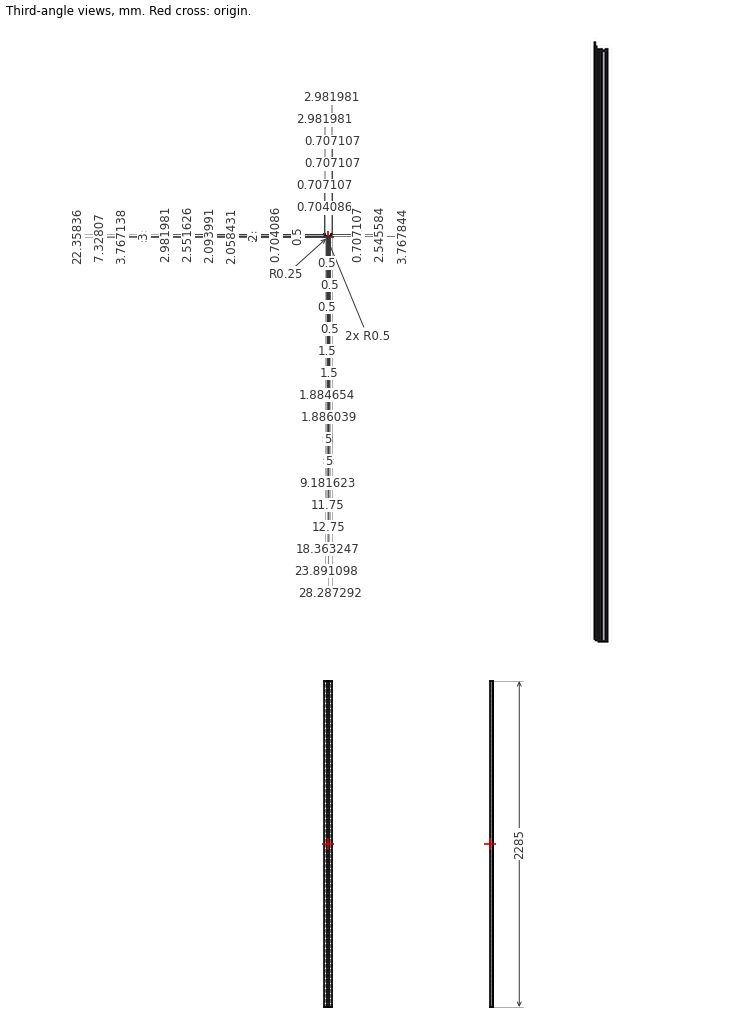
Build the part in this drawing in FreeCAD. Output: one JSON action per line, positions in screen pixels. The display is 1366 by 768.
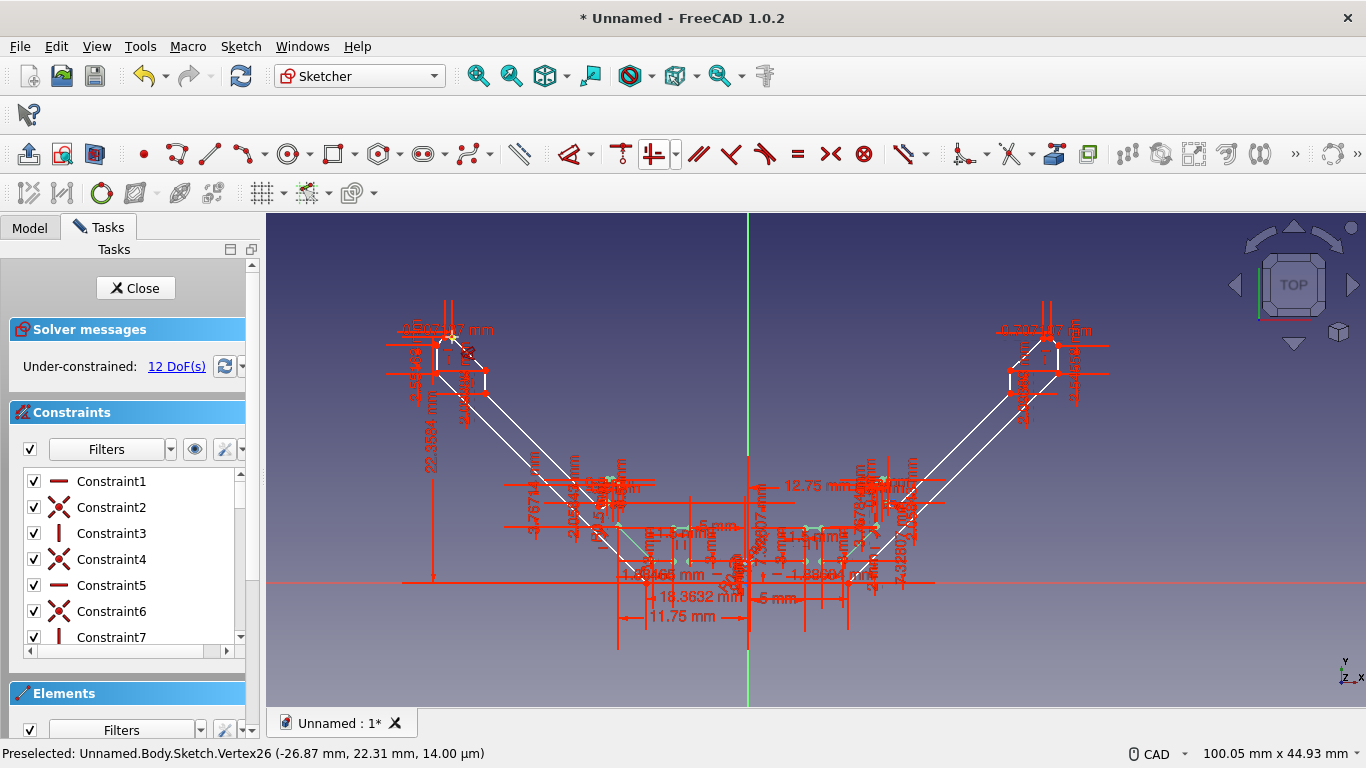
{"action": "left_click", "coordinate": [646, 583]}
{"action": "left_click", "coordinate": [697, 641]}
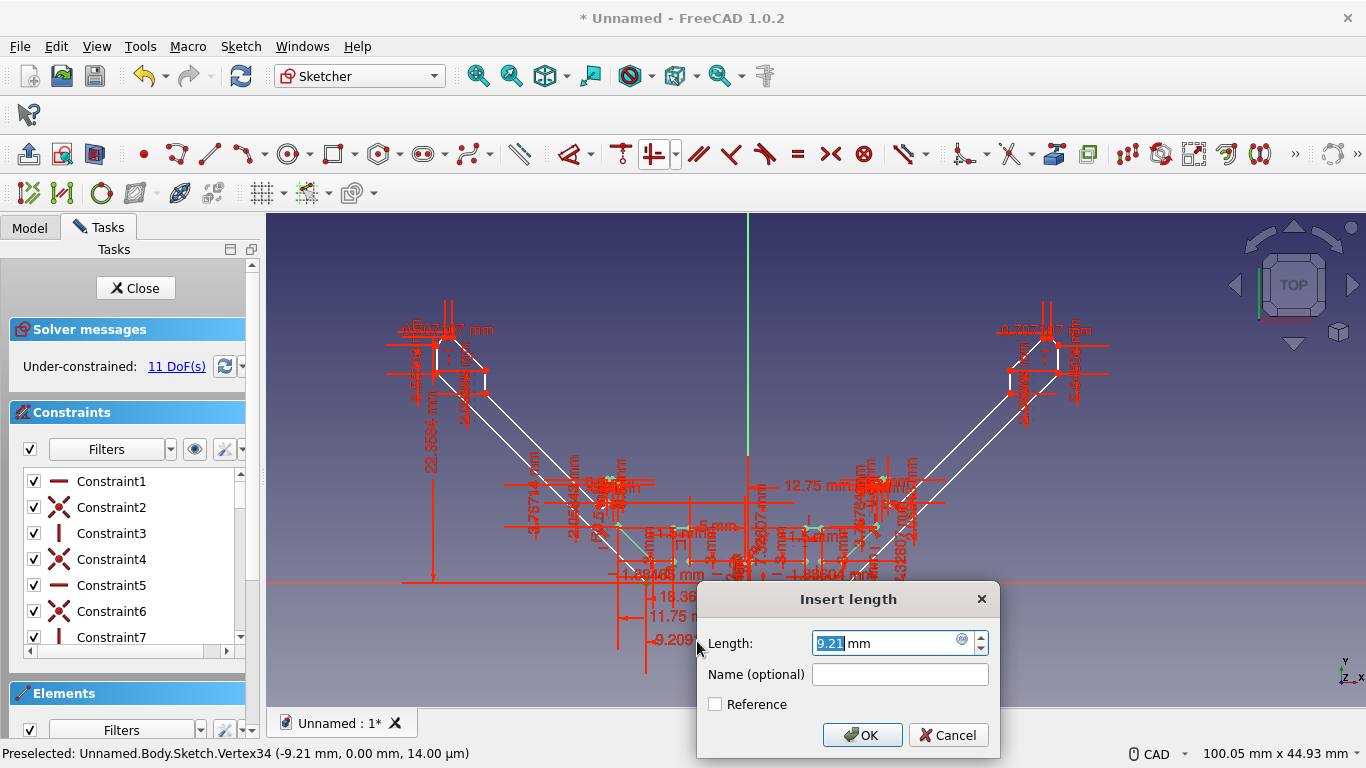
{"action": "type", "text": "9.181623"}
{"action": "key", "text": "Return"}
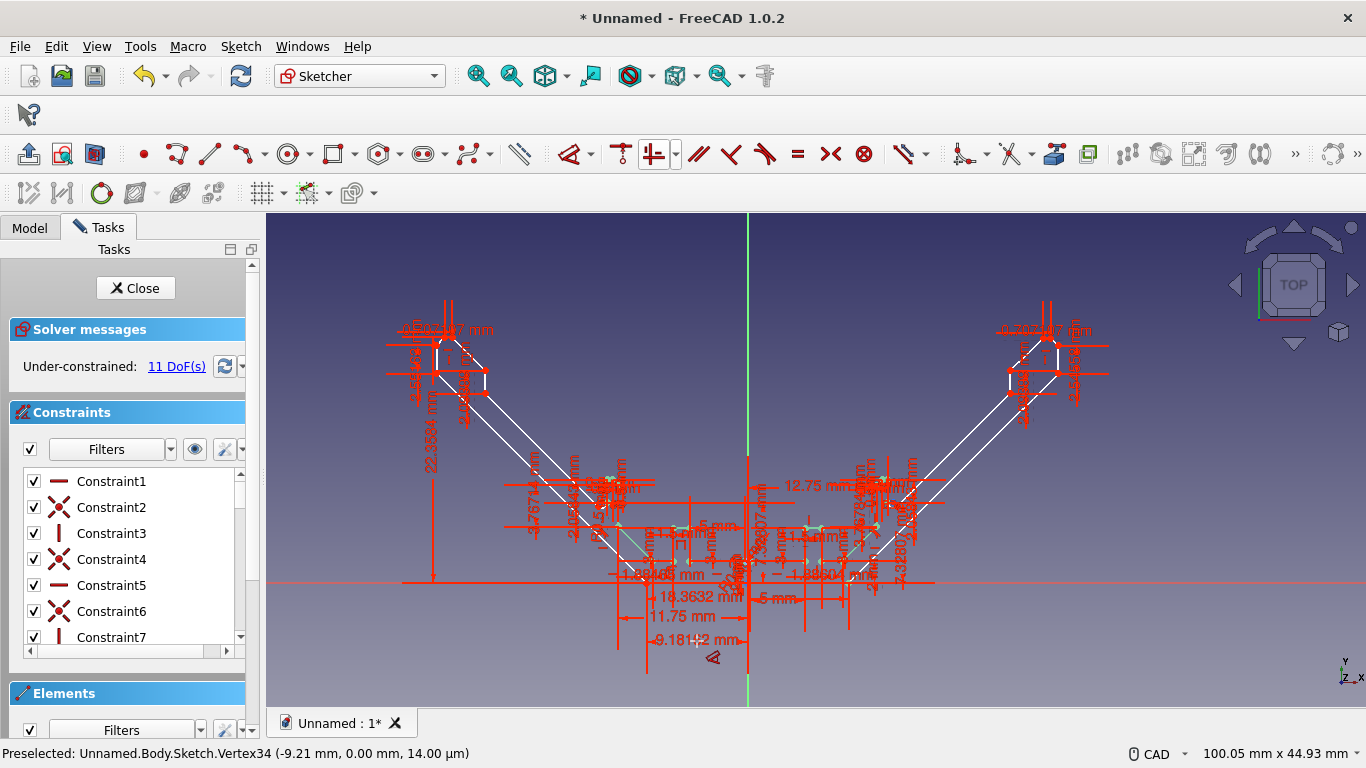
{"action": "scroll", "coordinate": [1051, 338], "scroll_direction": "up", "scroll_amount": 3}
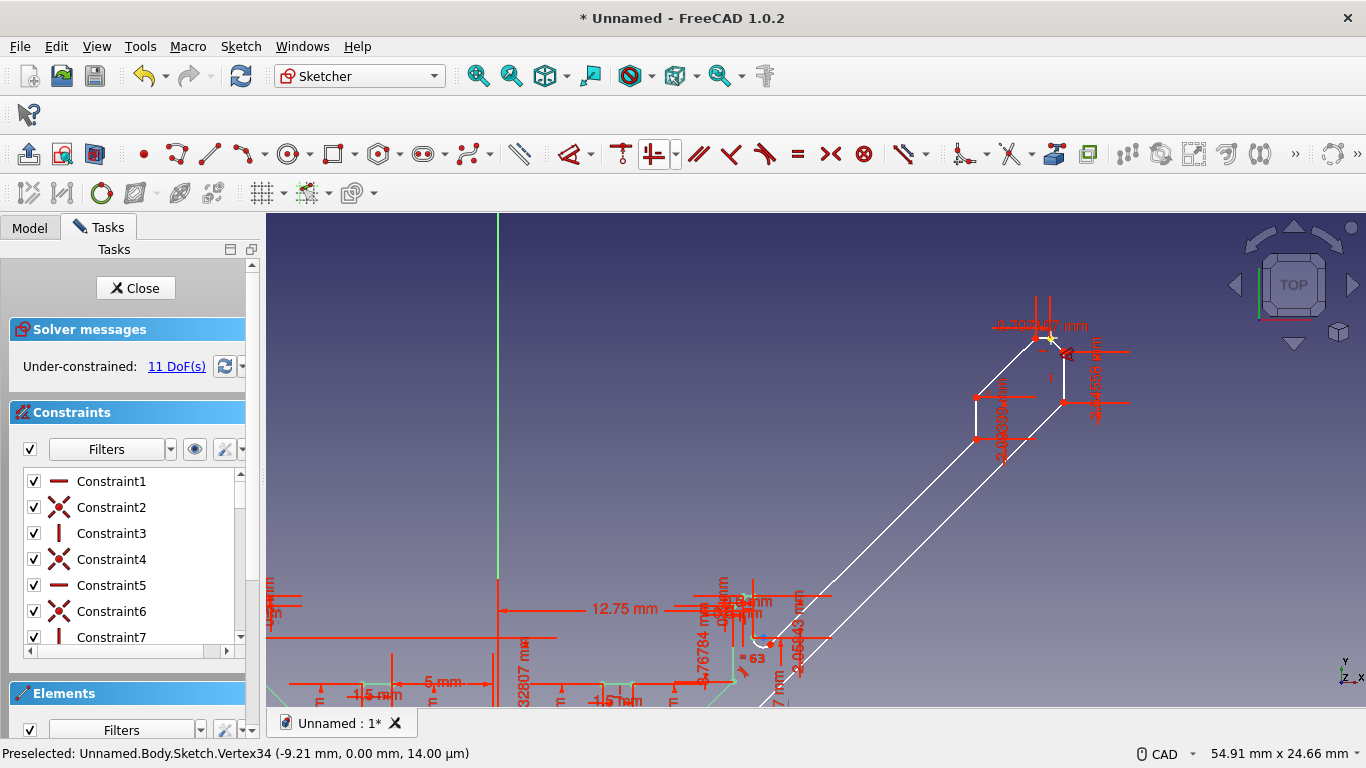
{"action": "left_click", "coordinate": [1050, 338]}
{"action": "left_click", "coordinate": [1084, 509]}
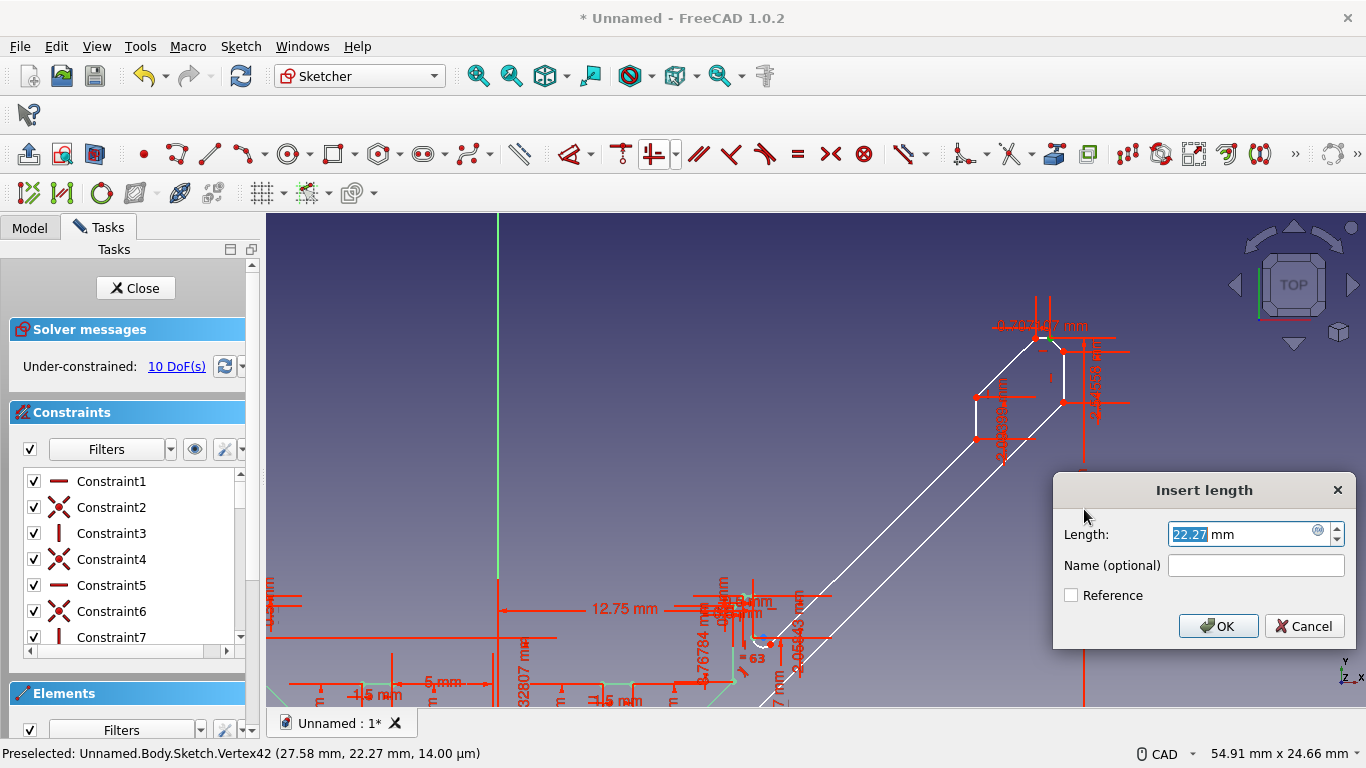
{"action": "type", "text": "22.35836"}
{"action": "key", "text": "Return"}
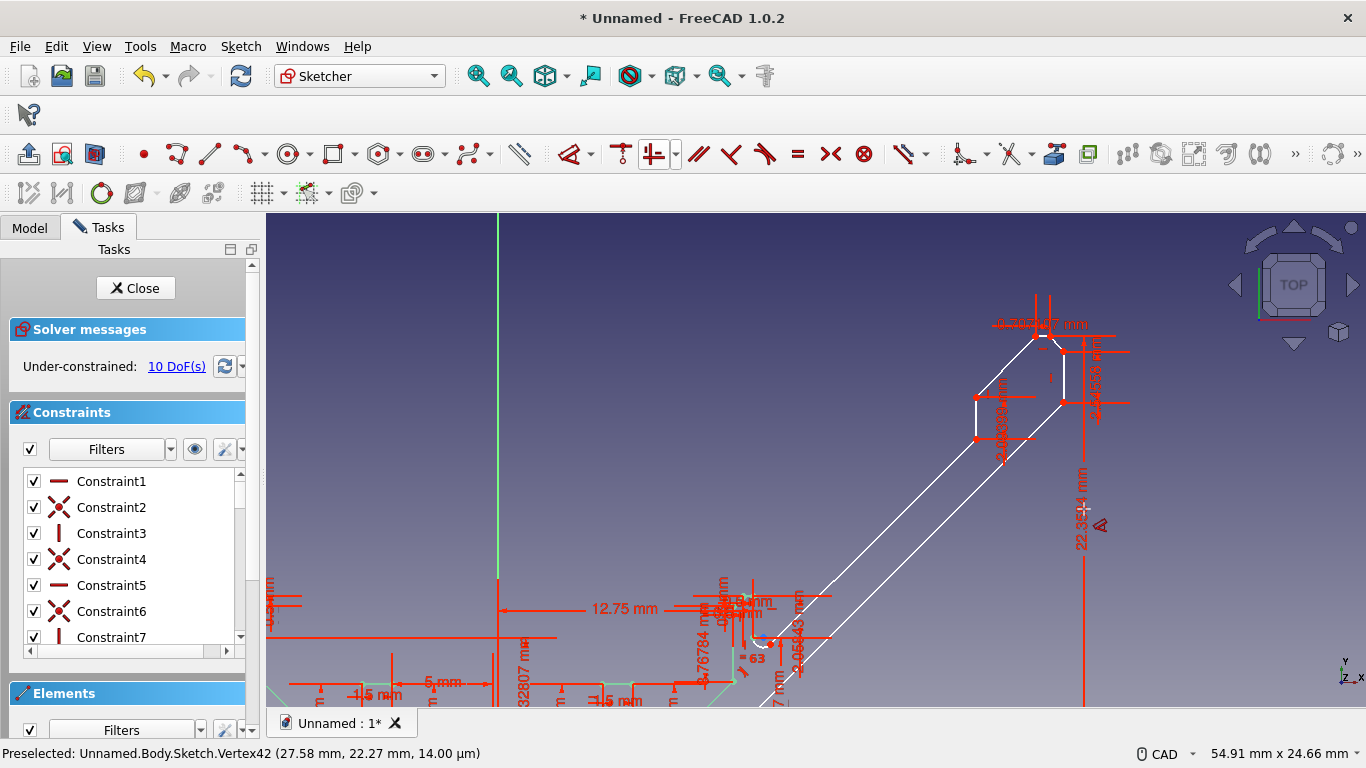
{"action": "scroll", "coordinate": [1051, 338], "scroll_direction": "down", "scroll_amount": 3}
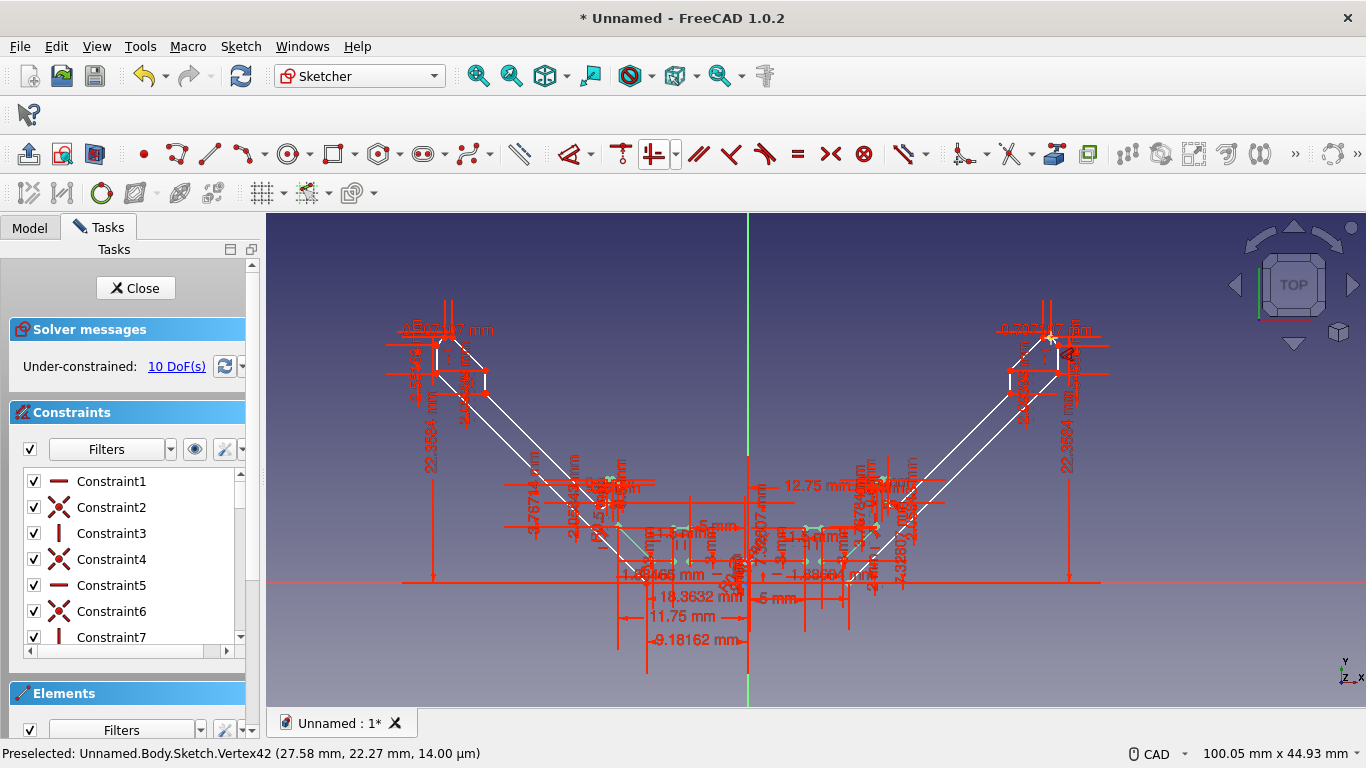
{"action": "left_click", "coordinate": [475, 361]}
{"action": "left_click", "coordinate": [469, 303]}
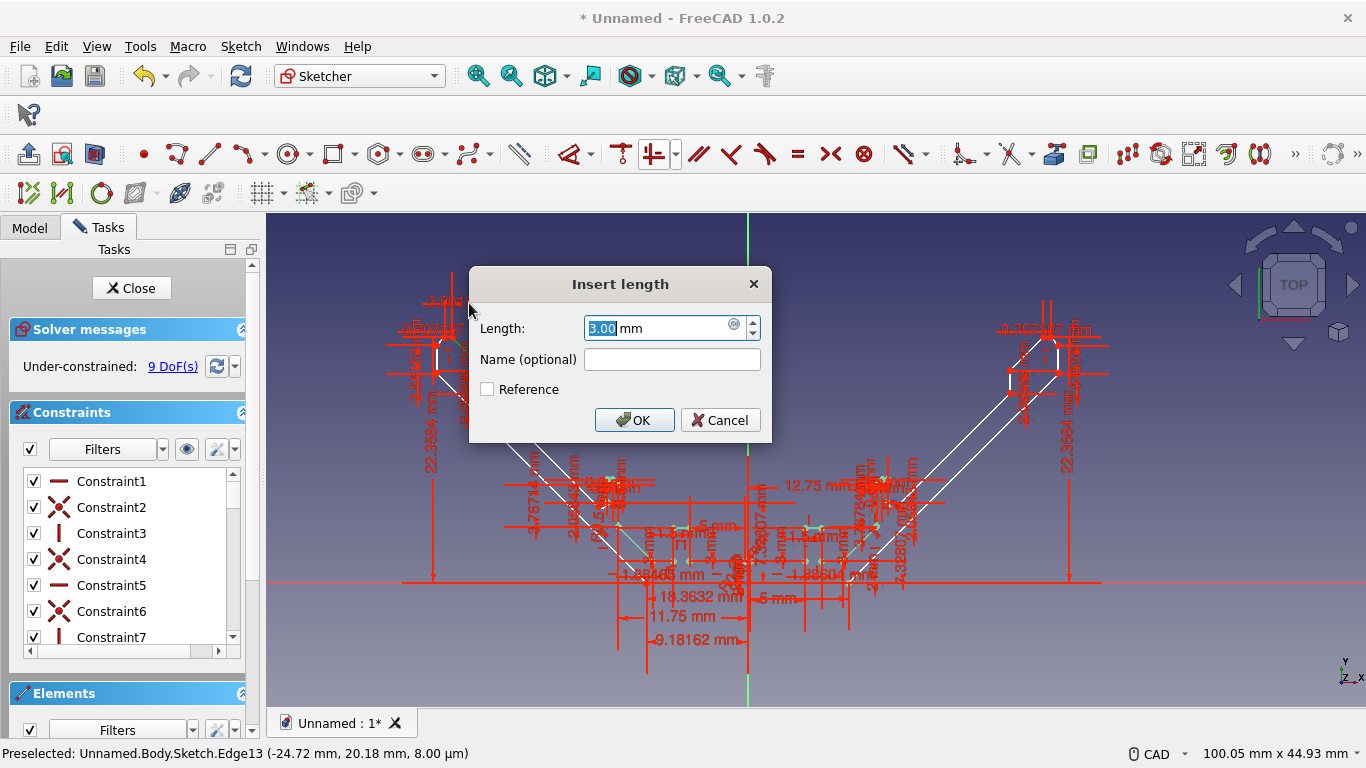
{"action": "type", "text": "2.981981"}
{"action": "key", "text": "Return"}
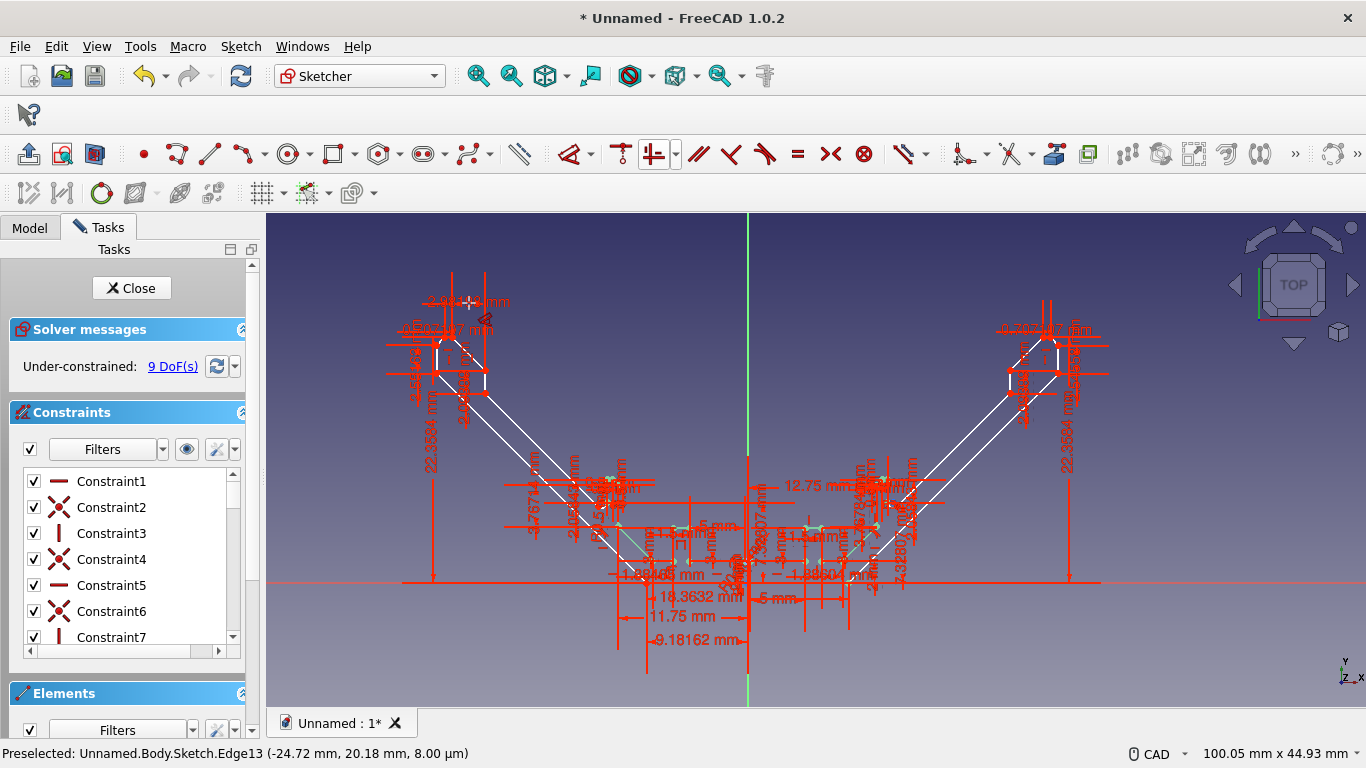
{"action": "left_click", "coordinate": [475, 361]}
{"action": "left_click", "coordinate": [519, 354]}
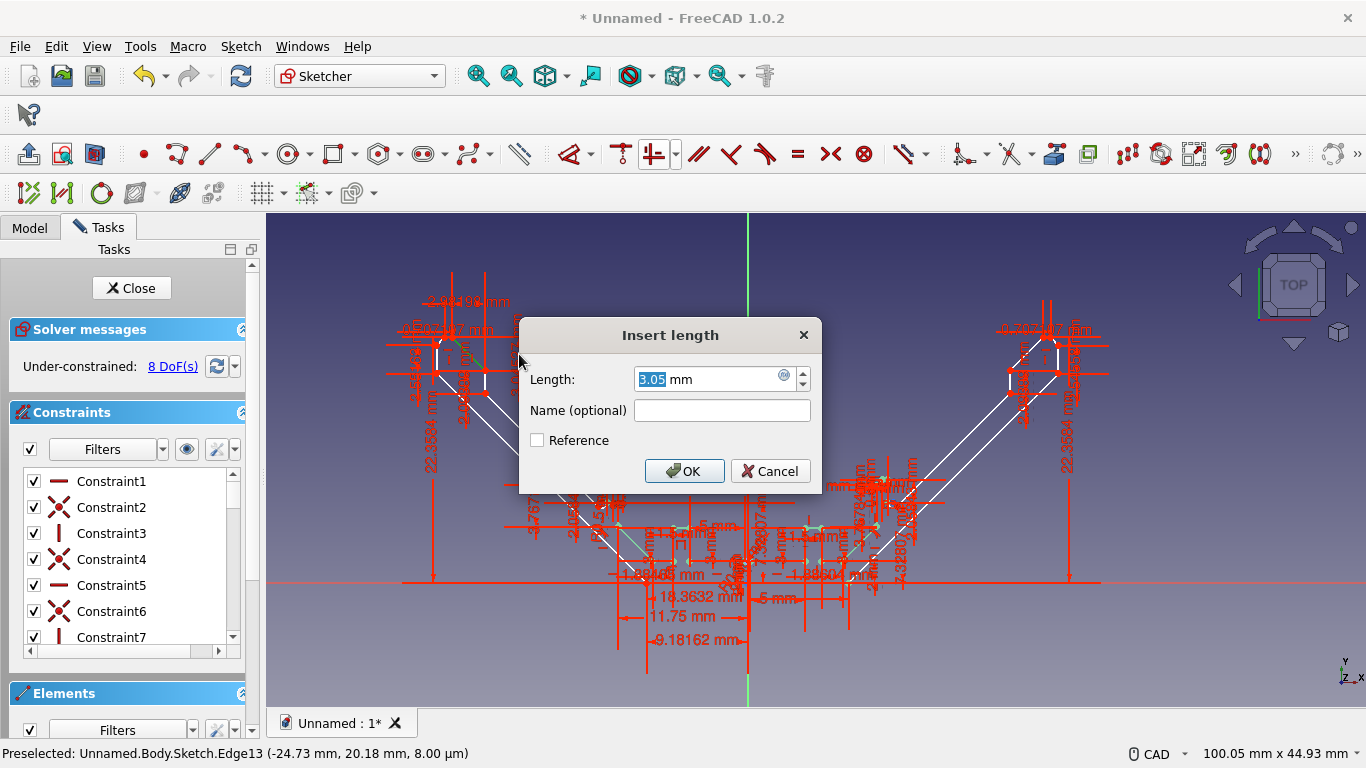
{"action": "type", "text": "2.981981"}
{"action": "key", "text": "Return"}